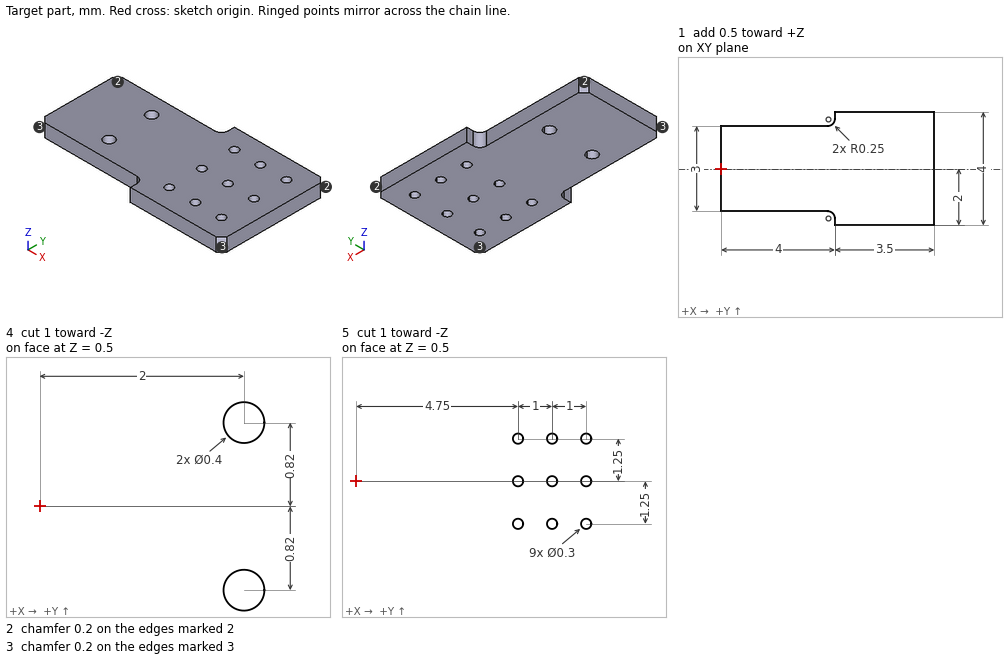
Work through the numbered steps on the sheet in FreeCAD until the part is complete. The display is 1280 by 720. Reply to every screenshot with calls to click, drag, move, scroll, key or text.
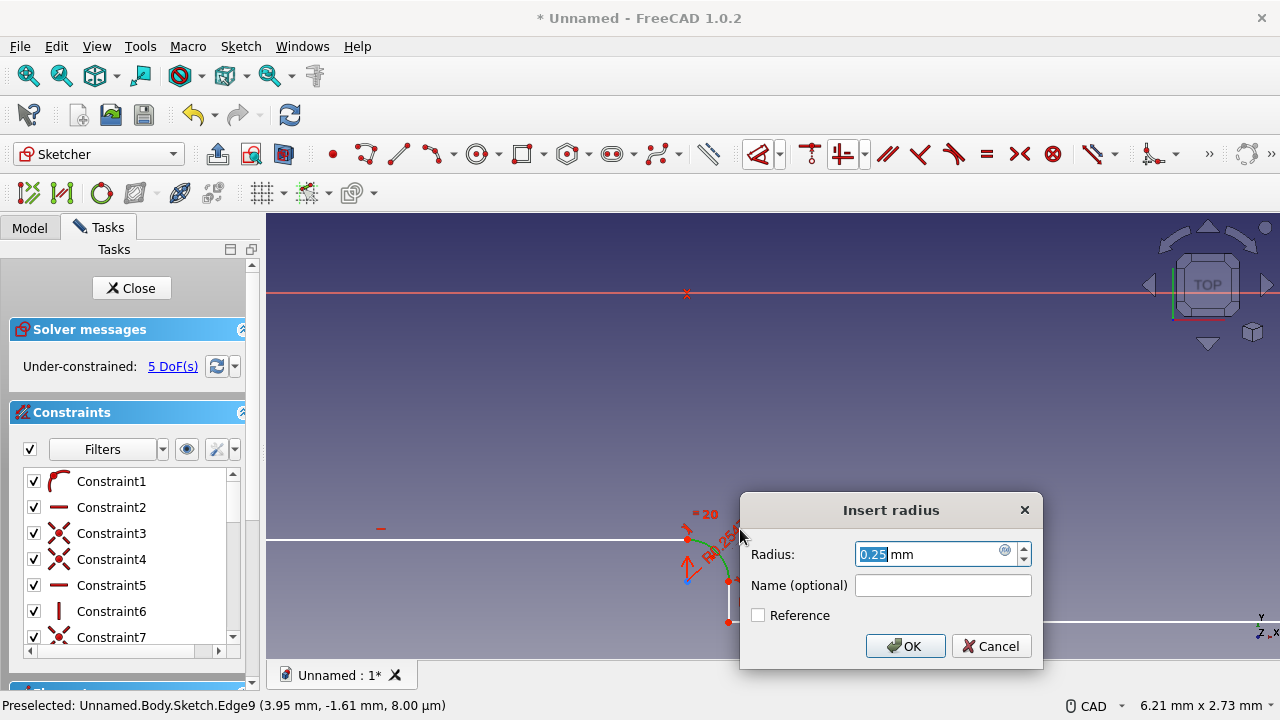
text(0.25)
key(Return)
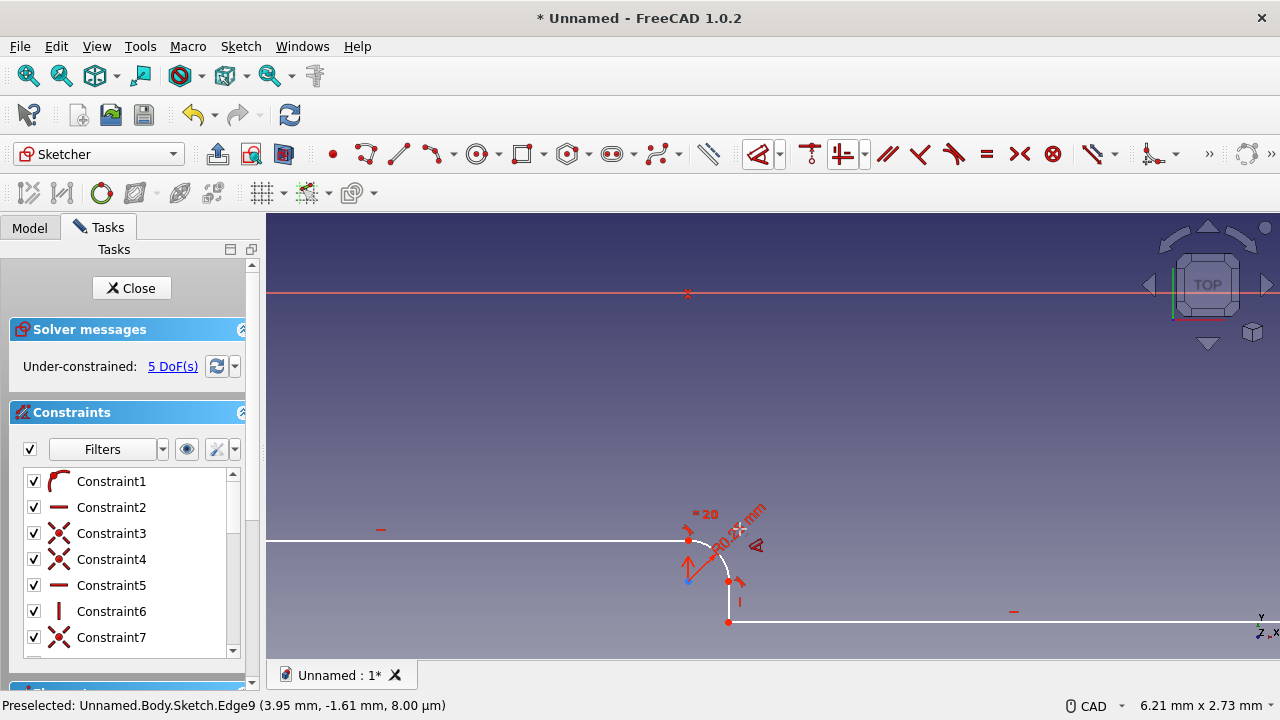
scroll(718, 552, down, 4)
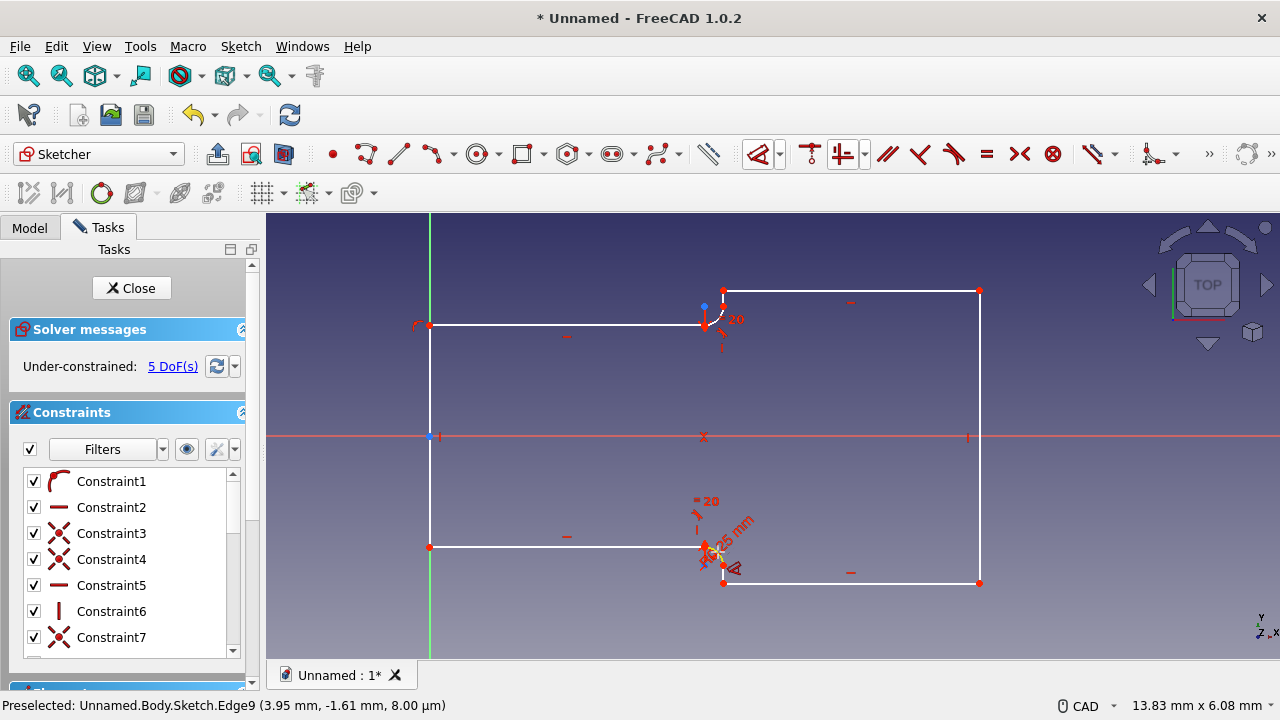
click(430, 392)
click(396, 385)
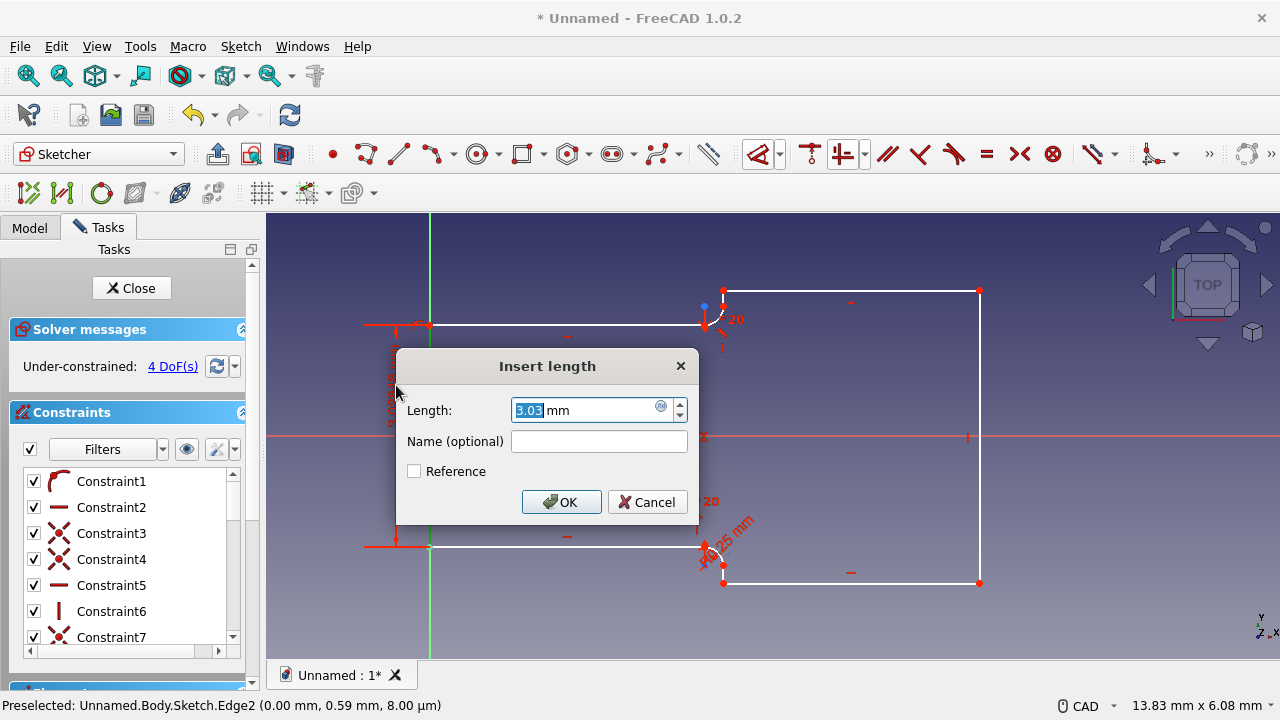
text(3)
key(Return)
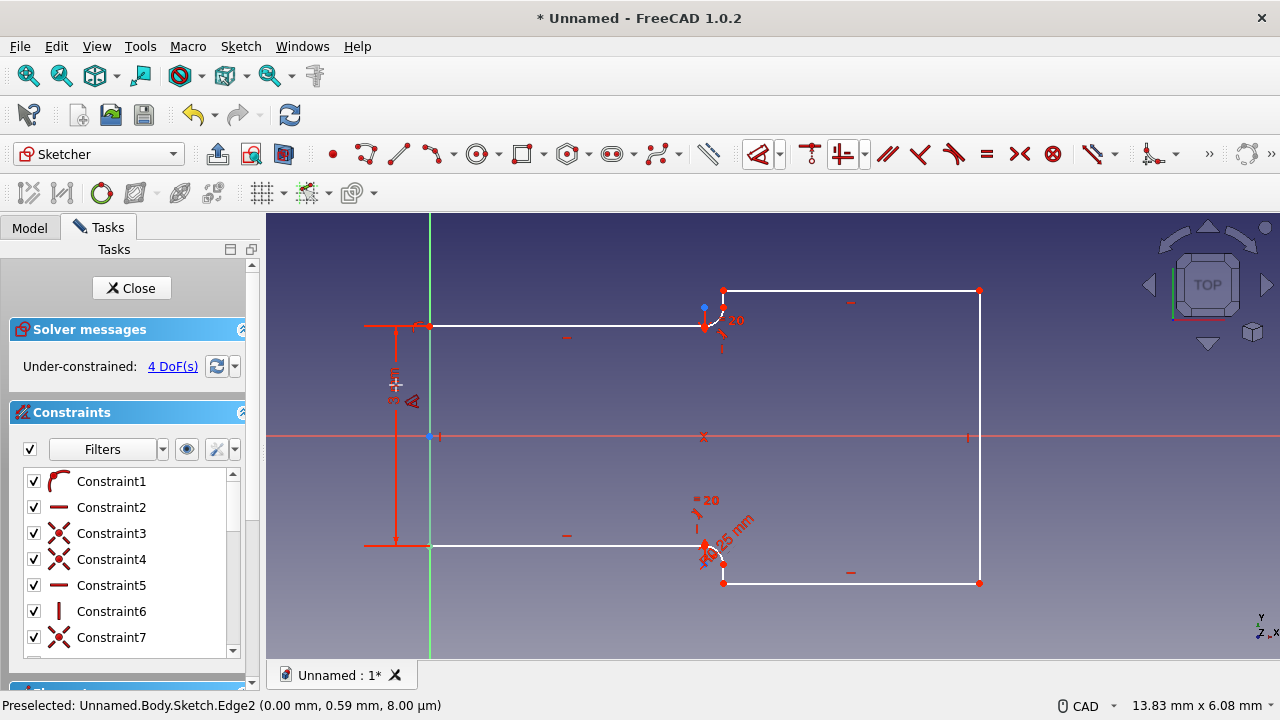
click(980, 496)
click(1014, 370)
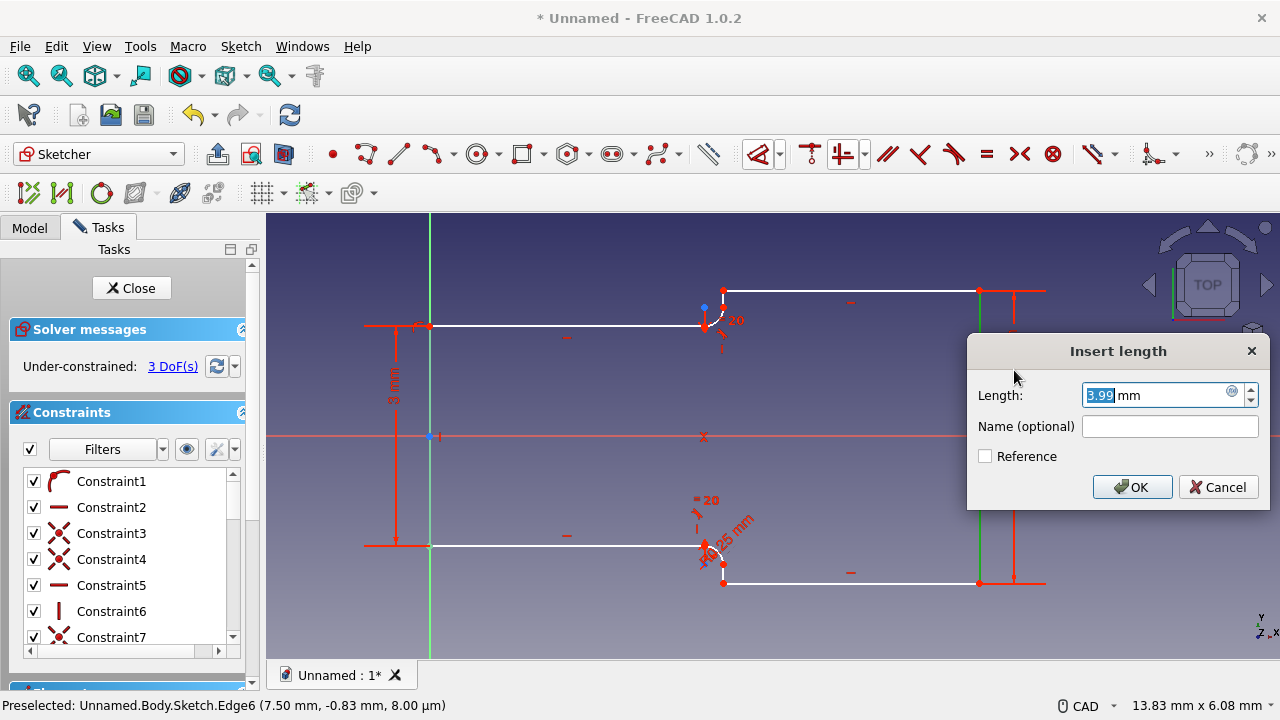
text(4)
key(Return)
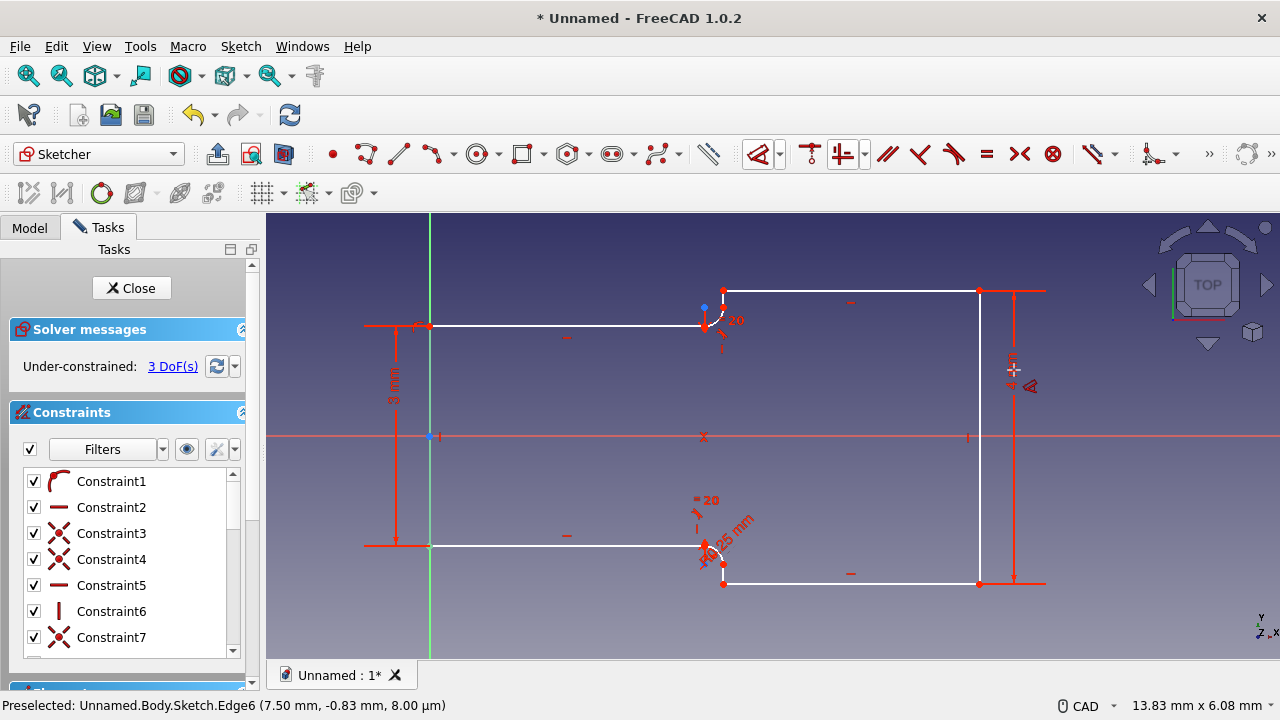
click(723, 565)
click(576, 599)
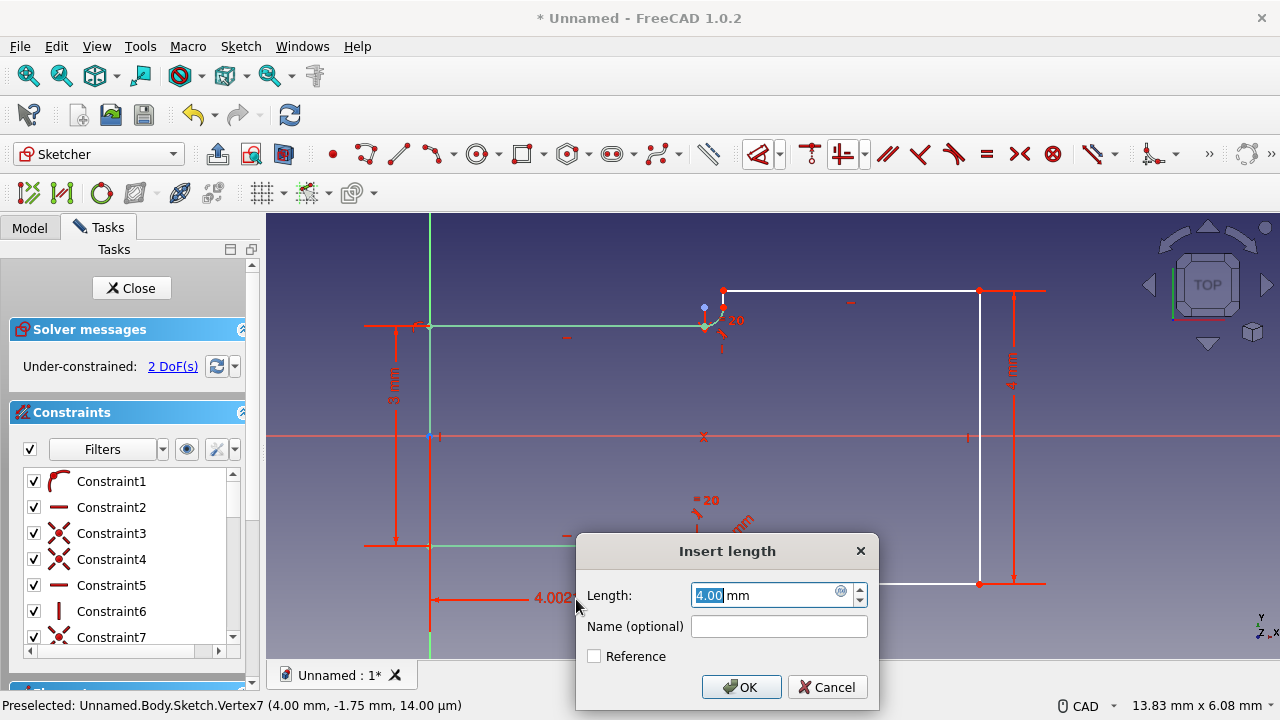
text(4)
key(Return)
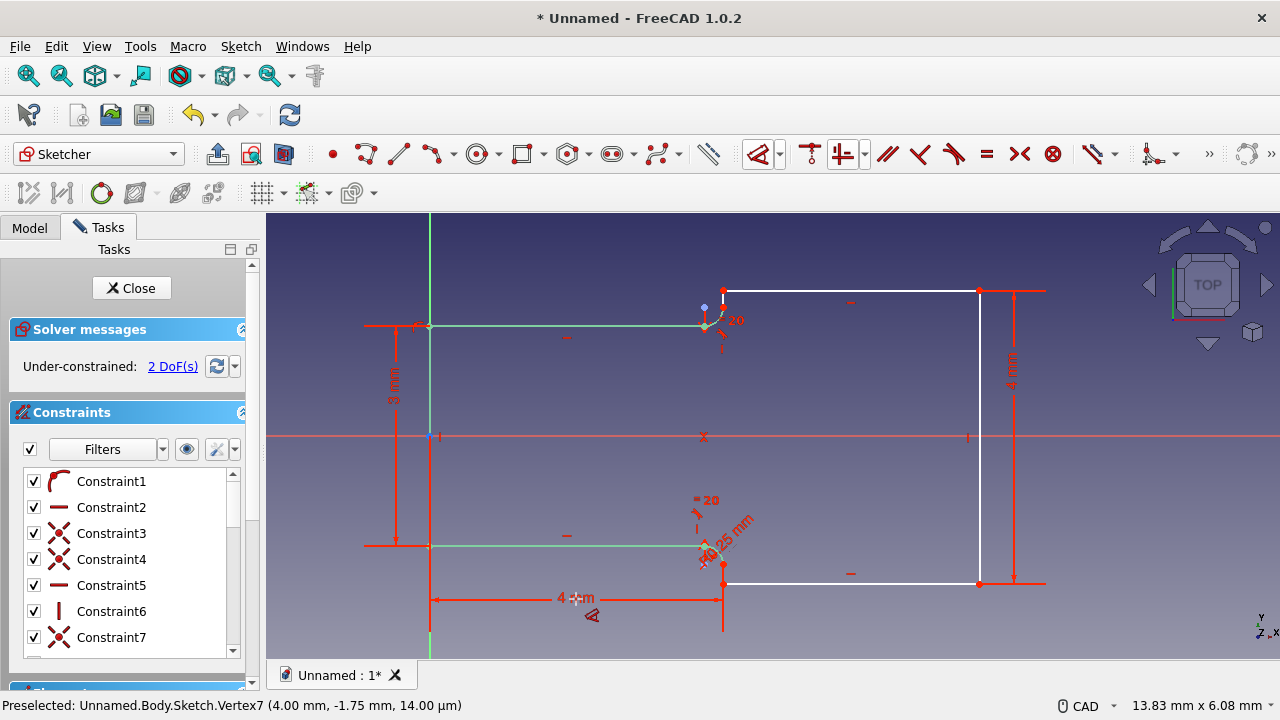
click(723, 584)
click(396, 510)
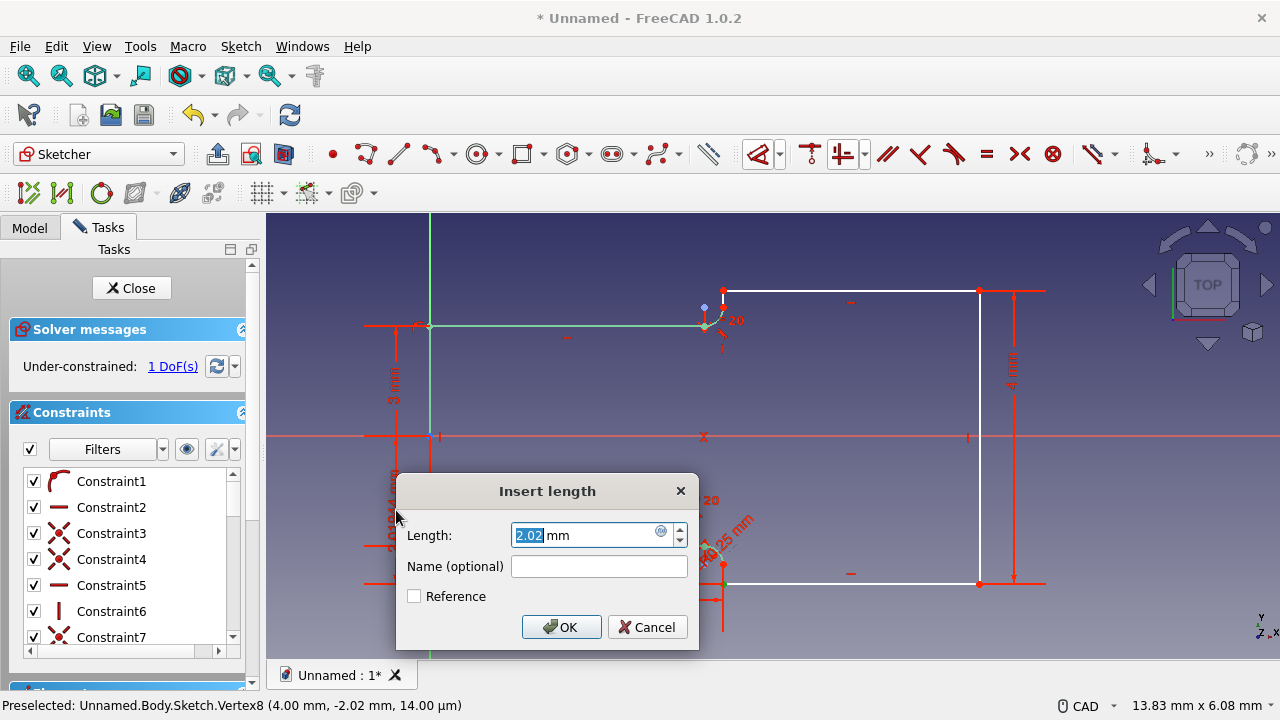
text(2)
key(Return)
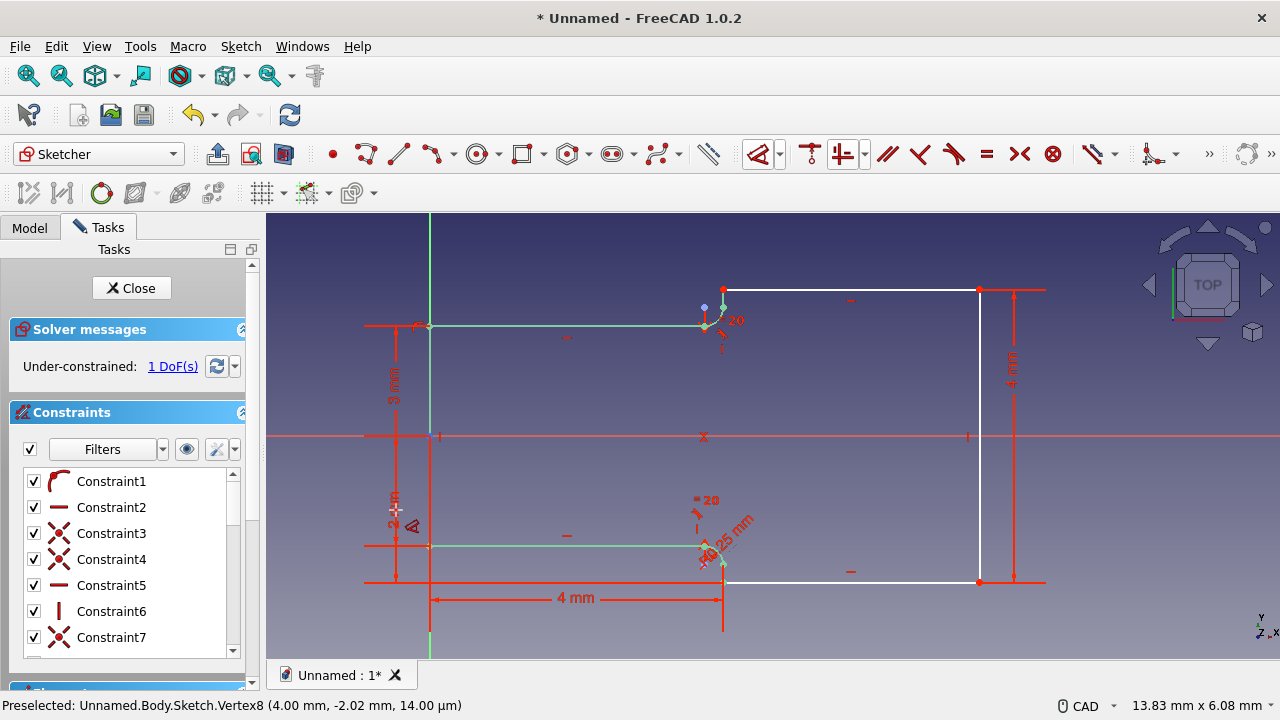
click(800, 583)
click(851, 617)